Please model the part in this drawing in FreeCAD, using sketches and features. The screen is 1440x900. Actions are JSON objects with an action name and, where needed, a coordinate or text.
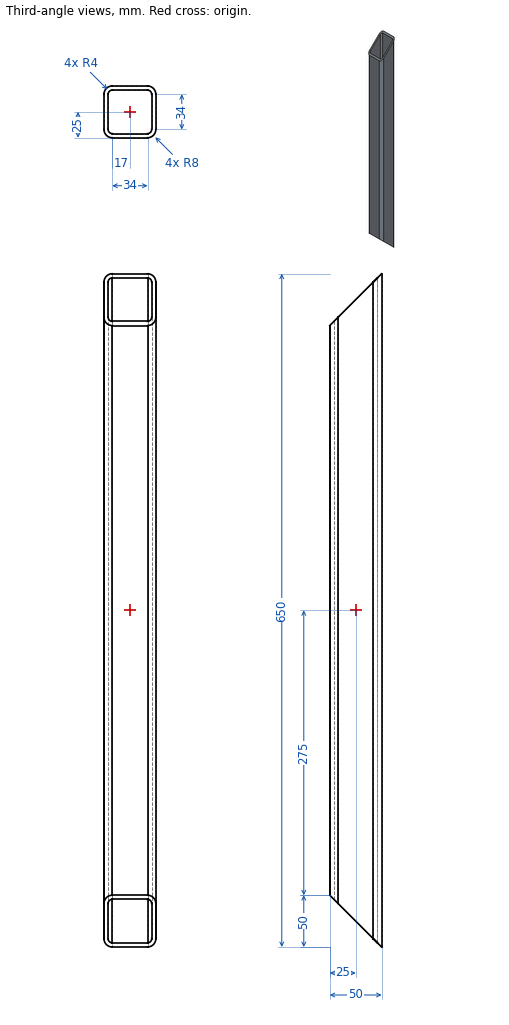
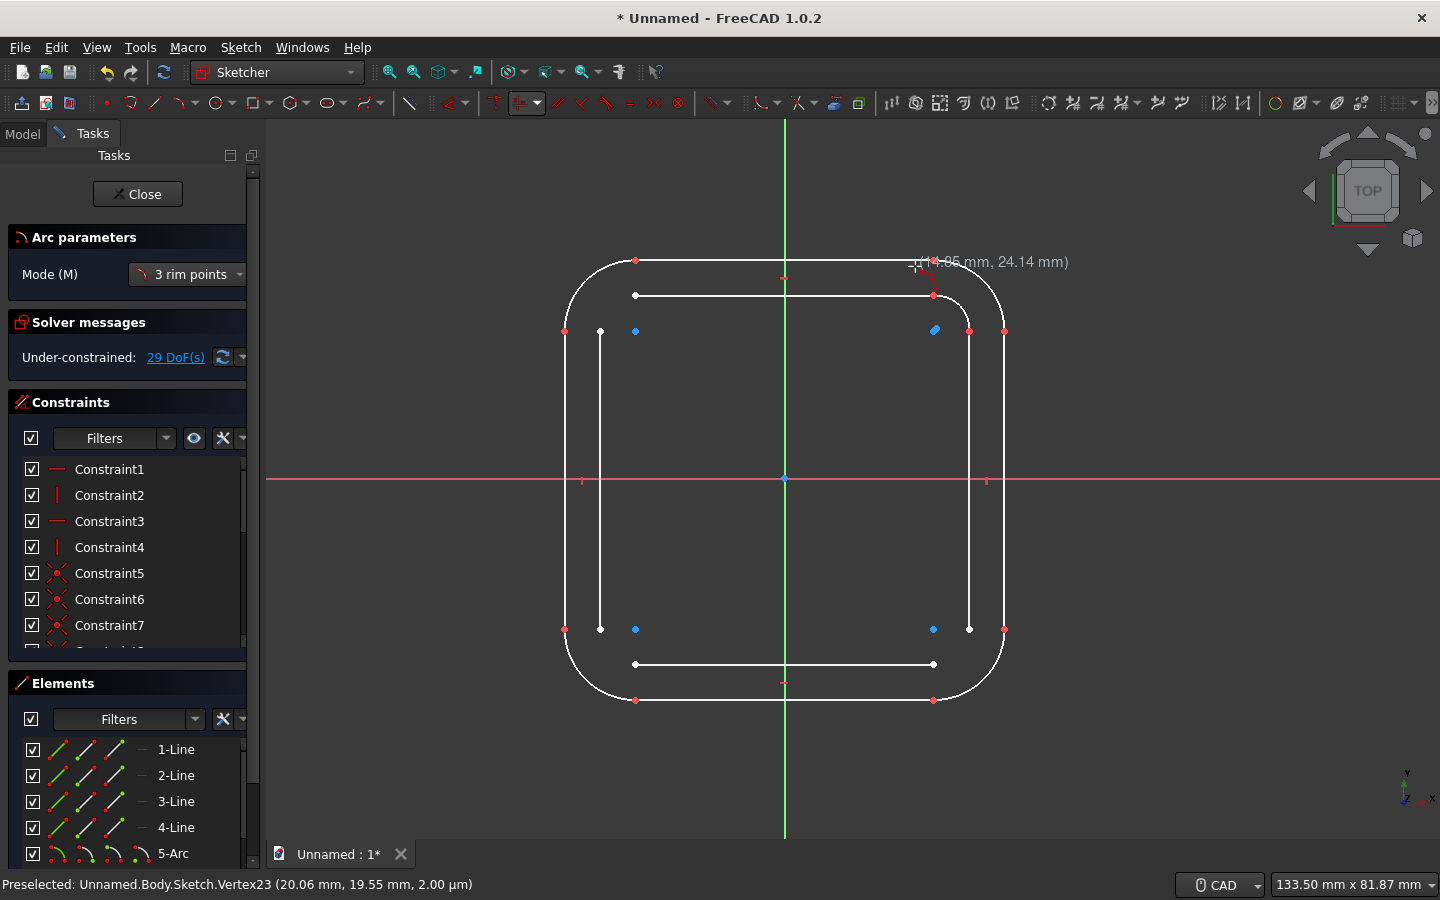
{"action": "left_click", "coordinate": [969, 629]}
{"action": "left_click", "coordinate": [934, 665]}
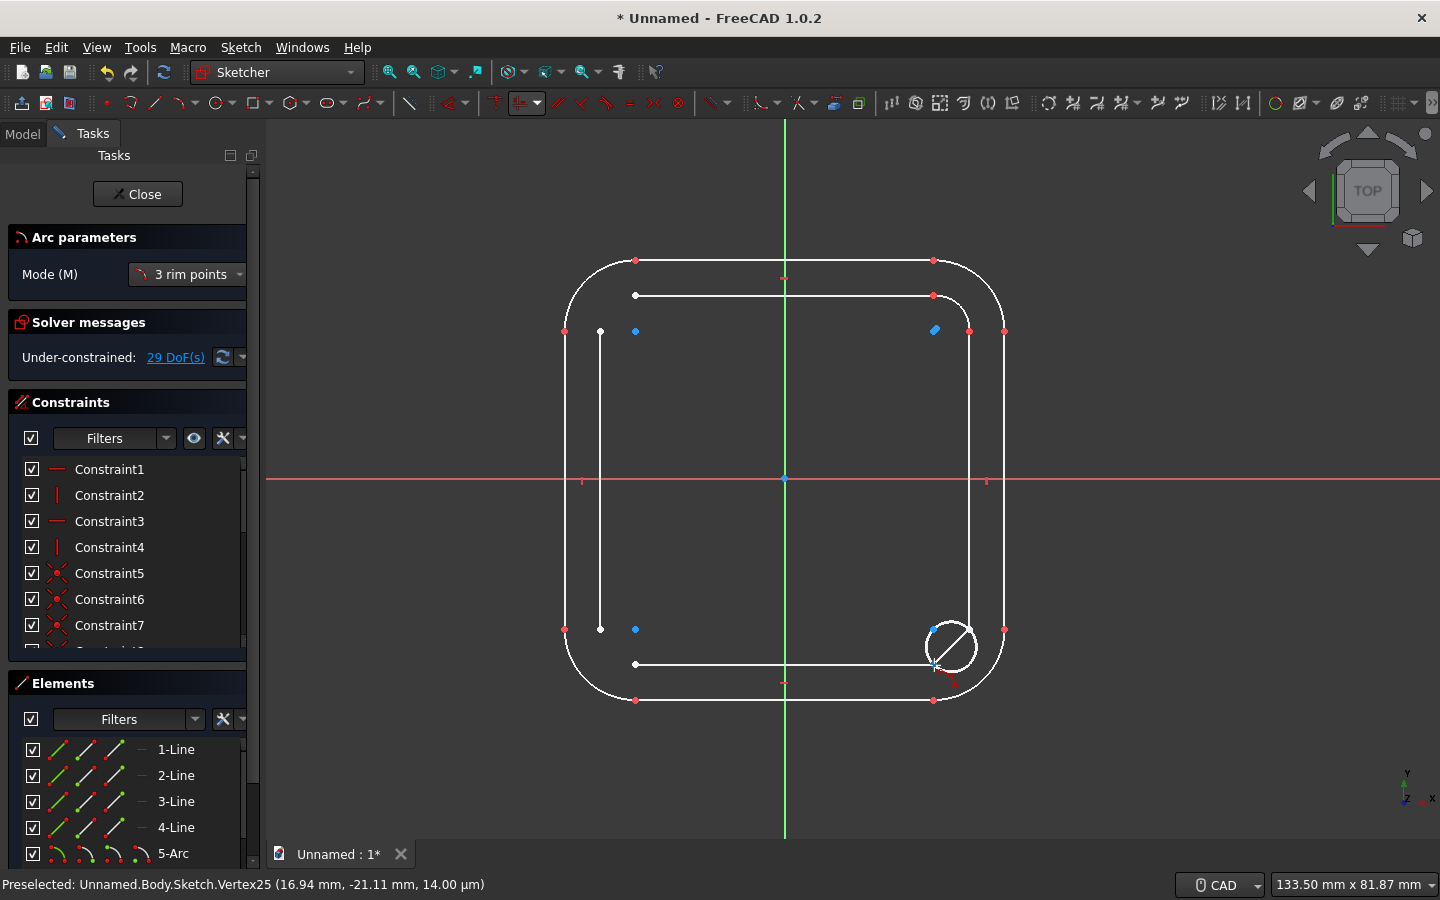
{"action": "scroll", "coordinate": [959, 653], "scroll_direction": "up", "scroll_amount": 3}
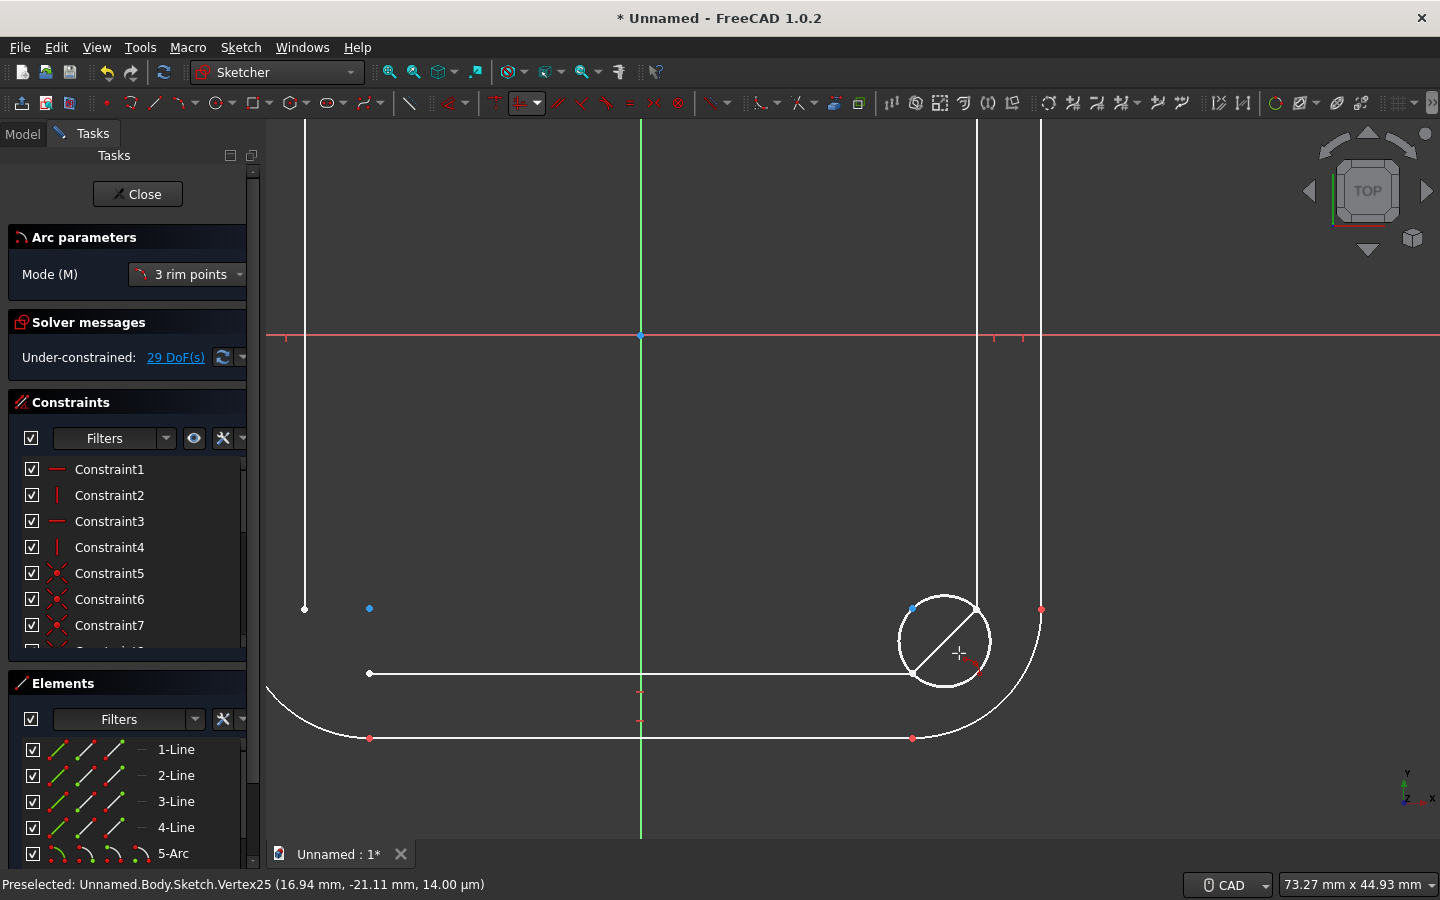
{"action": "left_click", "coordinate": [959, 653]}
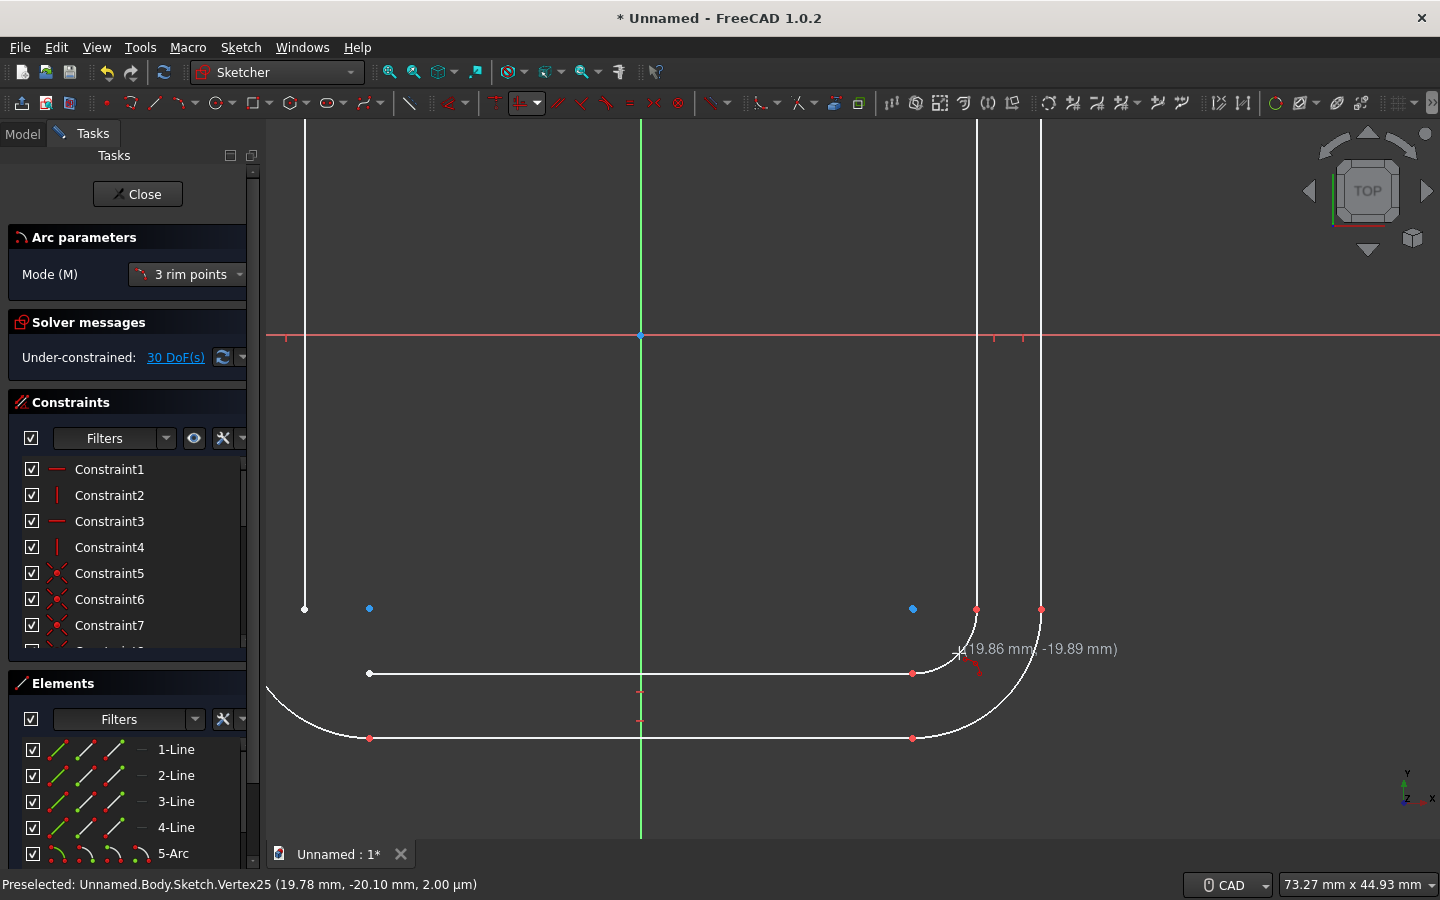
{"action": "left_click", "coordinate": [369, 674]}
{"action": "left_click", "coordinate": [305, 609]}
{"action": "left_click", "coordinate": [323, 653]}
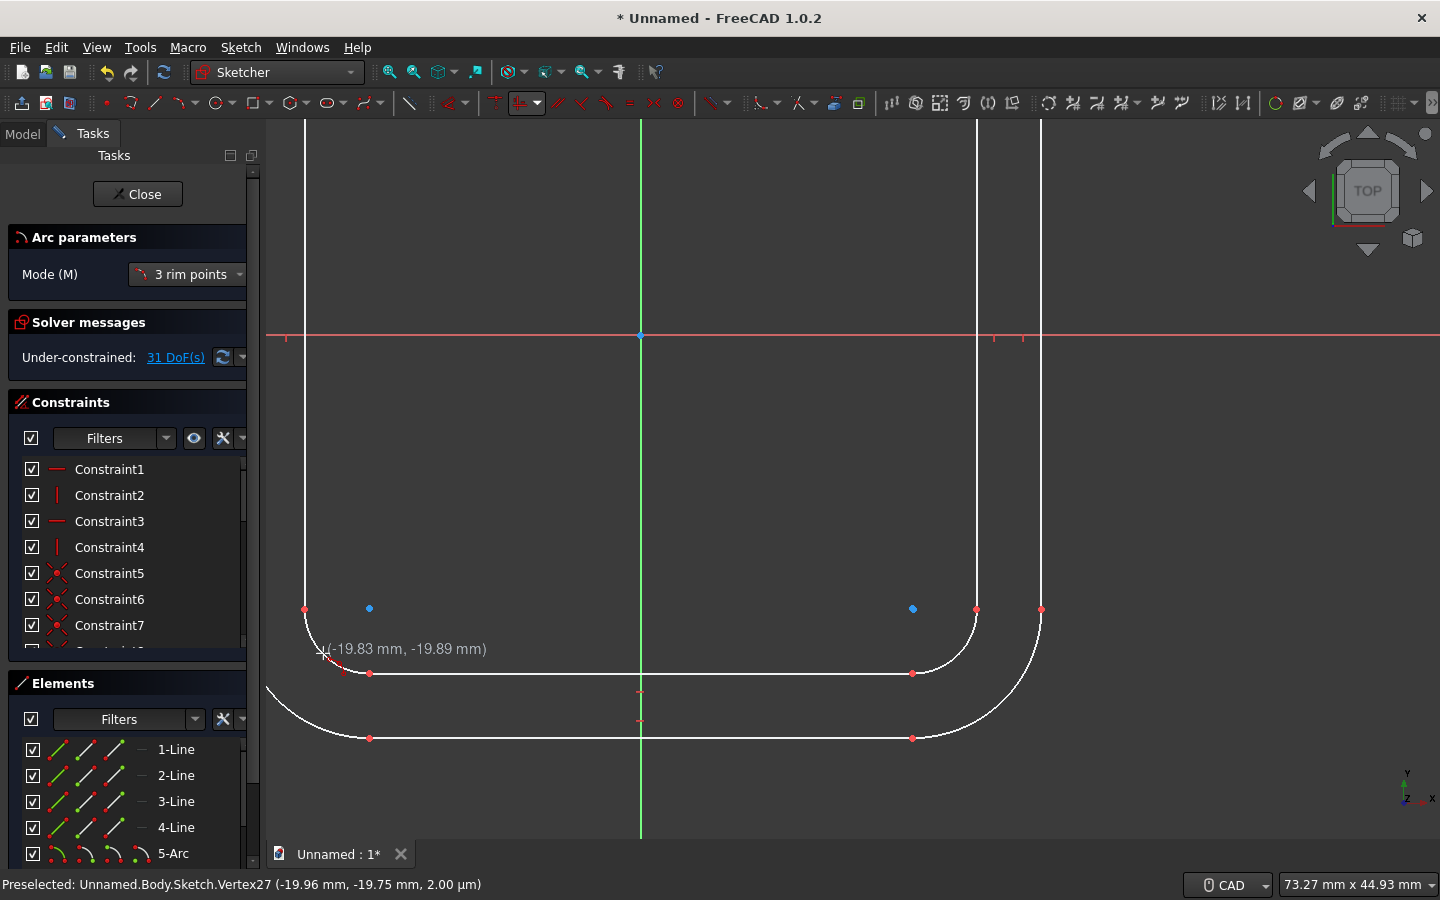
{"action": "scroll", "coordinate": [959, 654], "scroll_direction": "down", "scroll_amount": 3}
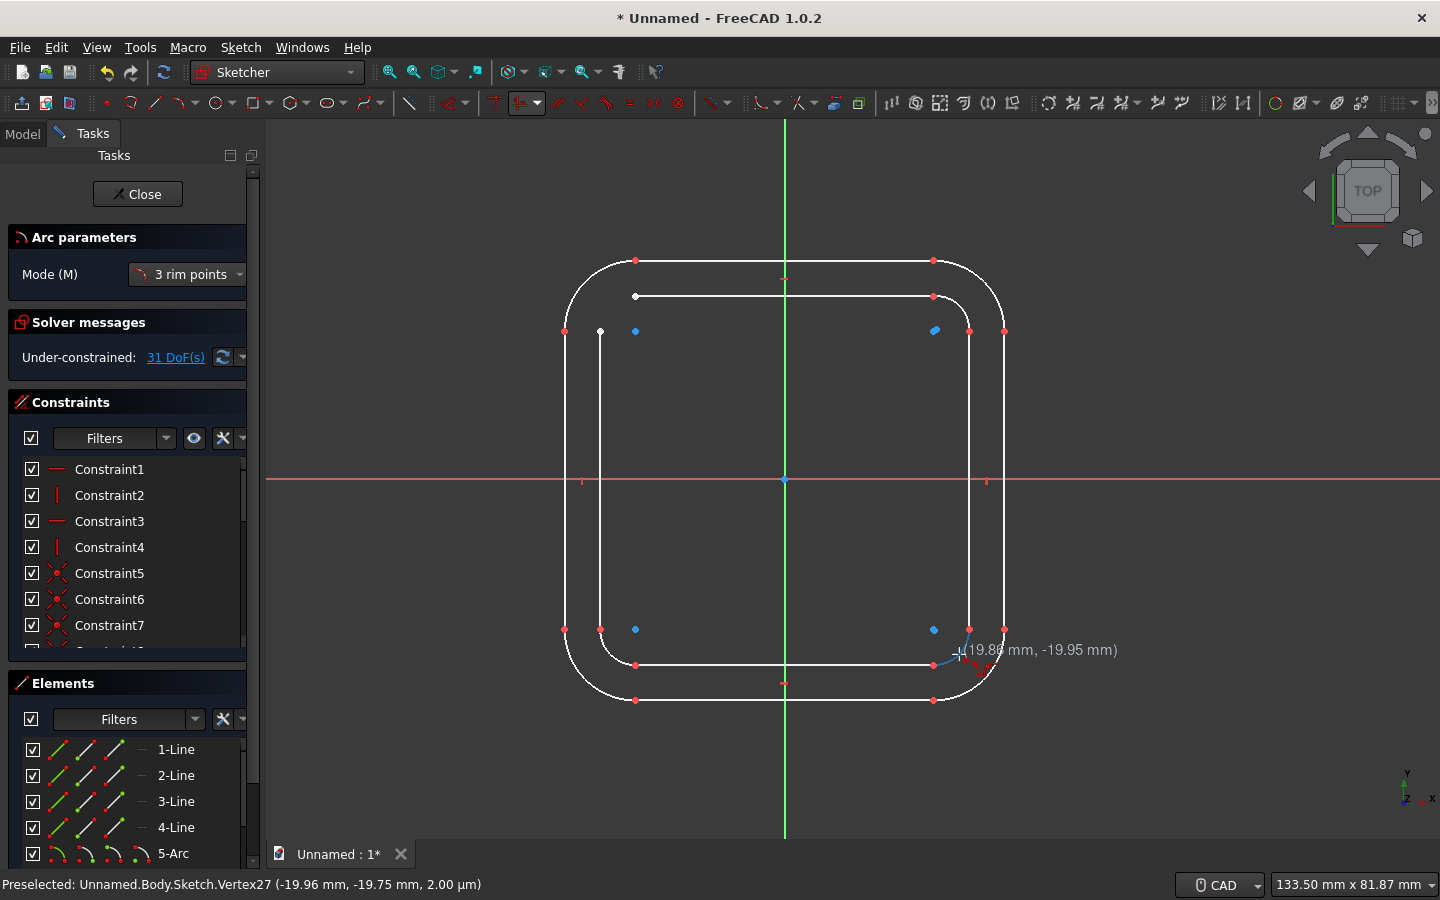
{"action": "left_click", "coordinate": [600, 332]}
{"action": "left_click", "coordinate": [636, 296]}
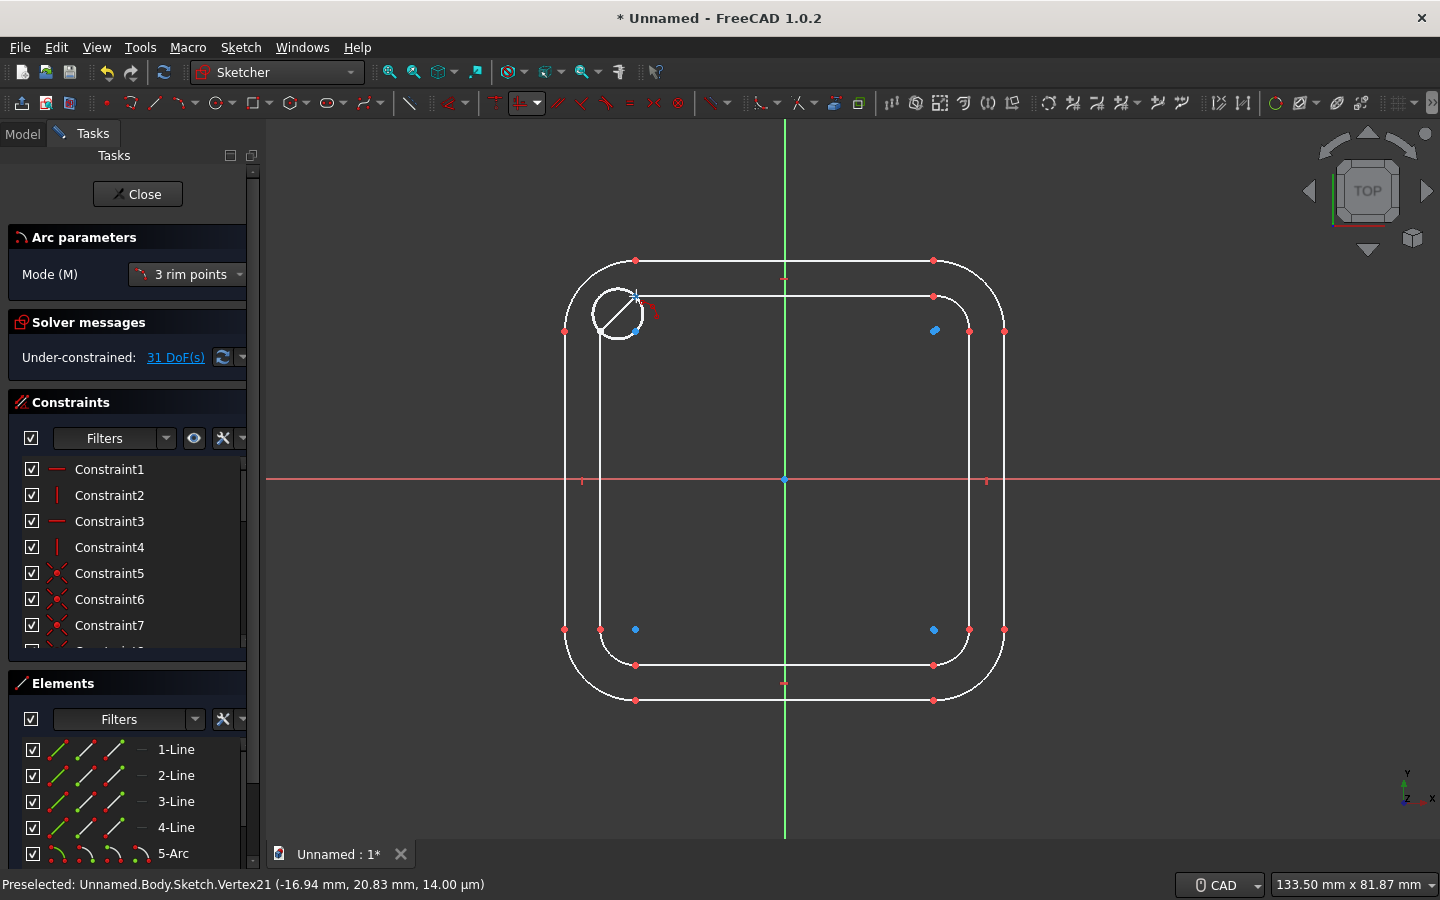
{"action": "scroll", "coordinate": [610, 305], "scroll_direction": "up", "scroll_amount": 3}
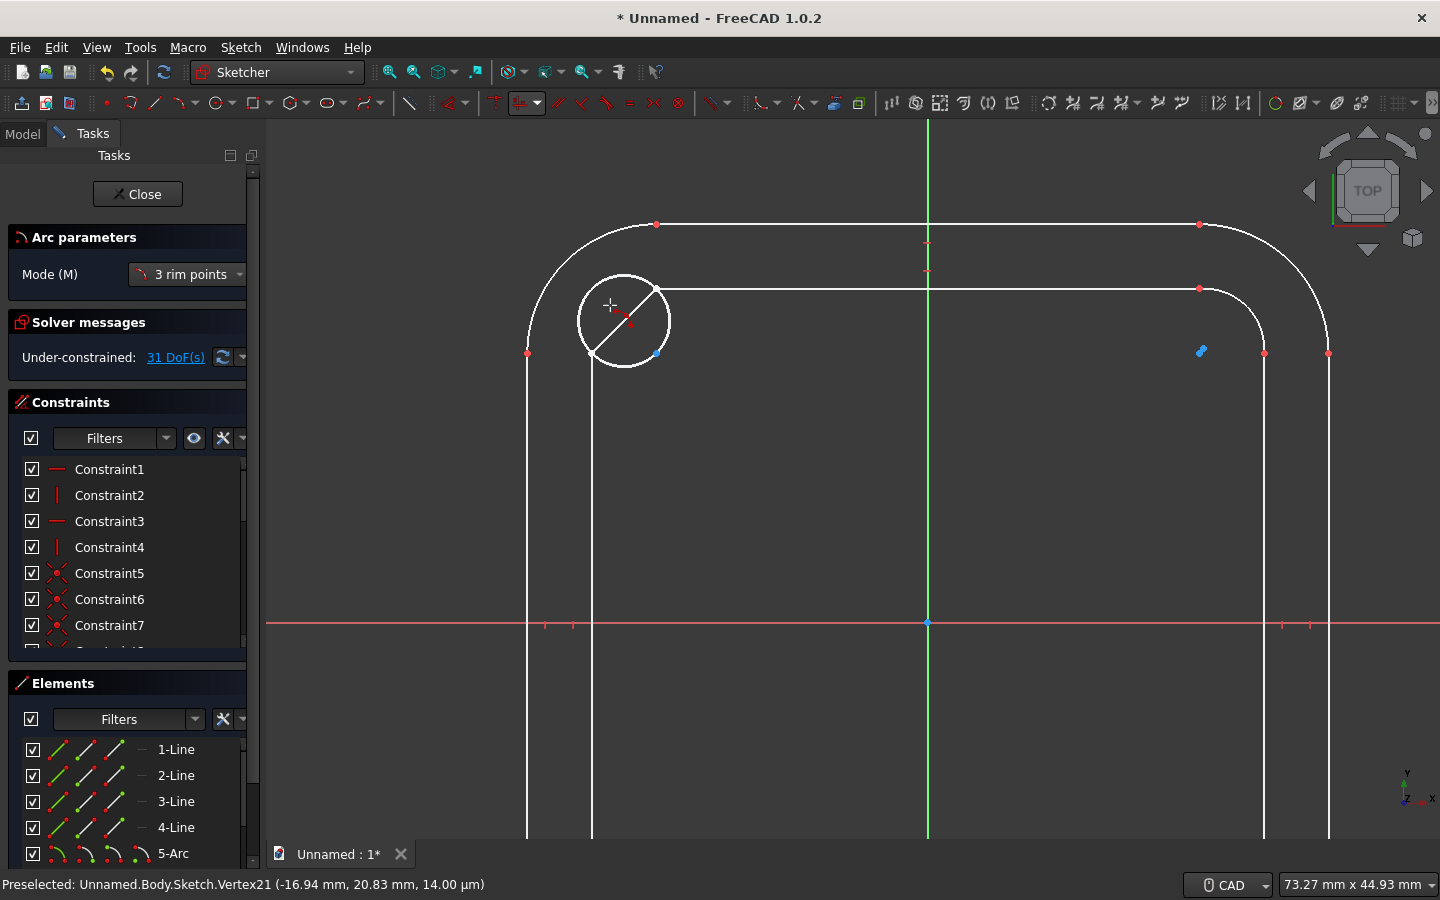
{"action": "left_click", "coordinate": [610, 305]}
{"action": "key", "text": "Escape"}